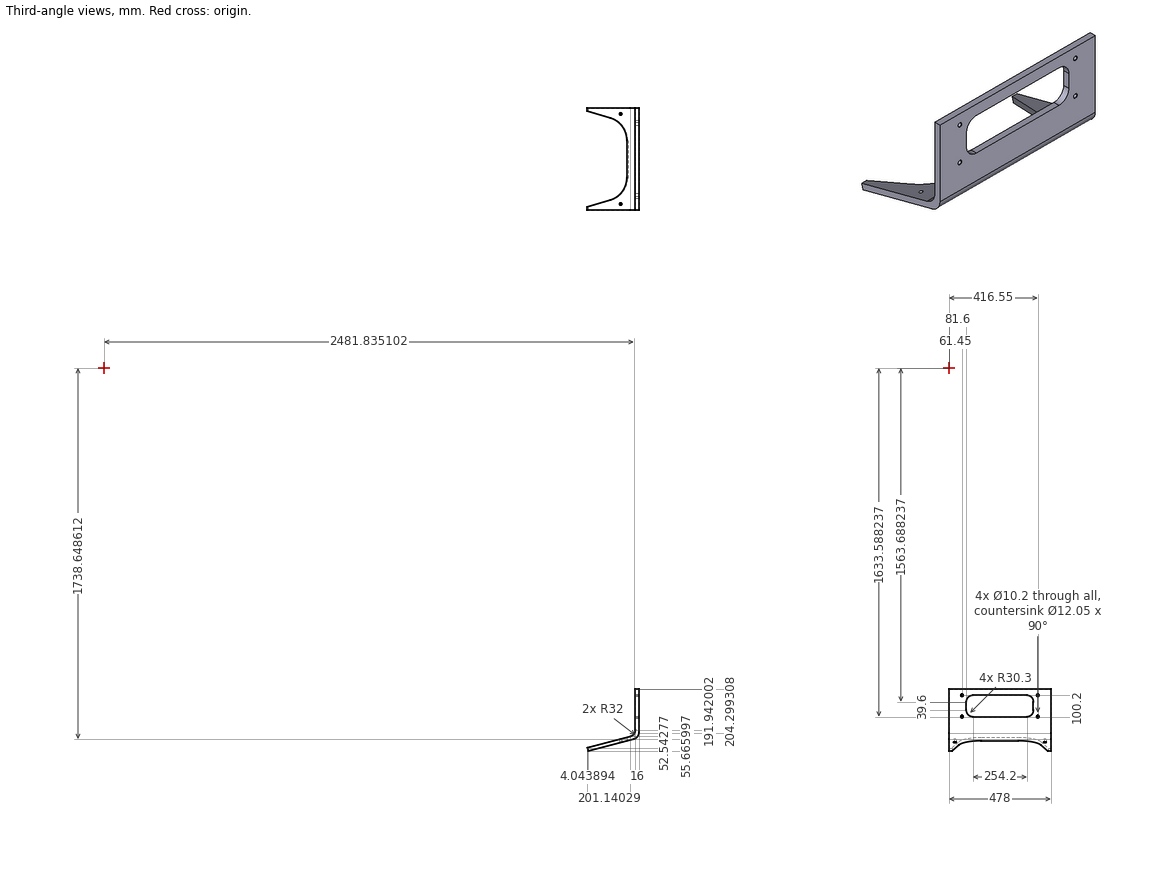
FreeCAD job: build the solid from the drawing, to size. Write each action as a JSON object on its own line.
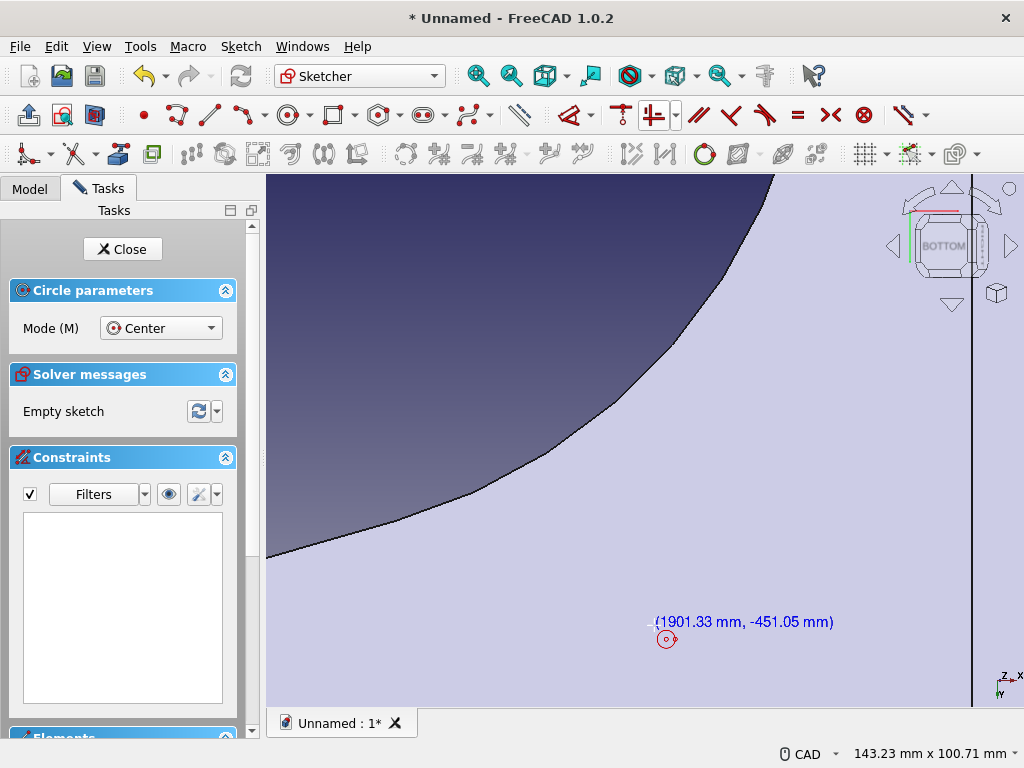
{"action": "scroll", "coordinate": [565, 587], "scroll_direction": "down", "scroll_amount": 10}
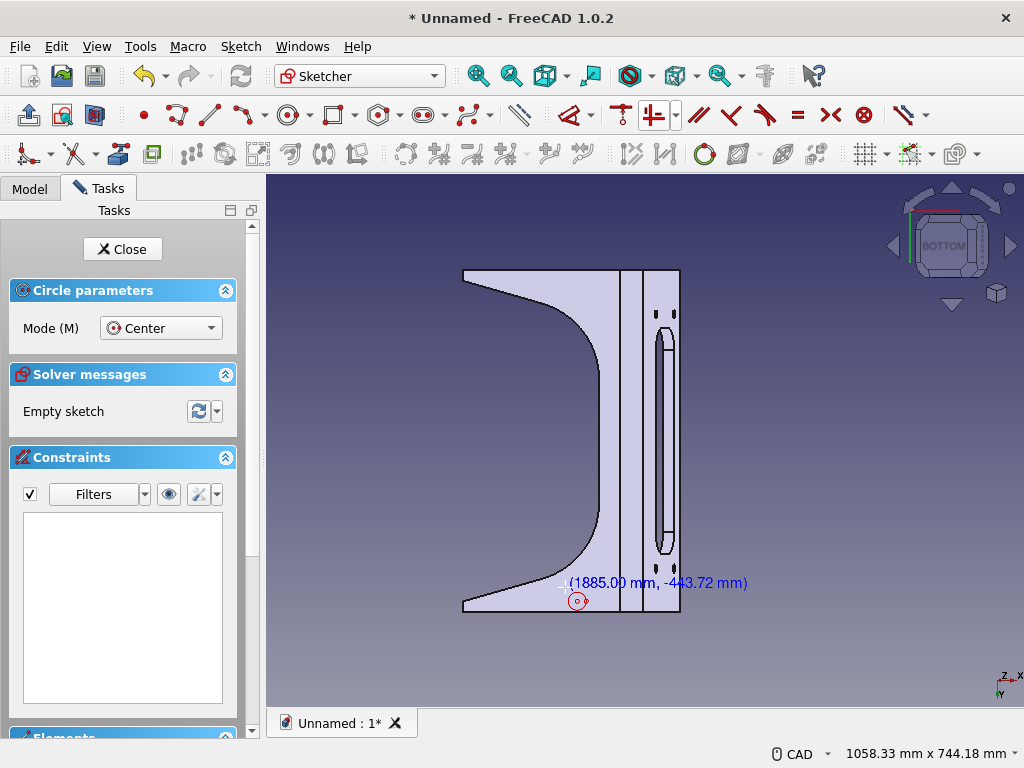
{"action": "left_click", "coordinate": [577, 592]}
{"action": "mouse_move", "coordinate": [580, 590]}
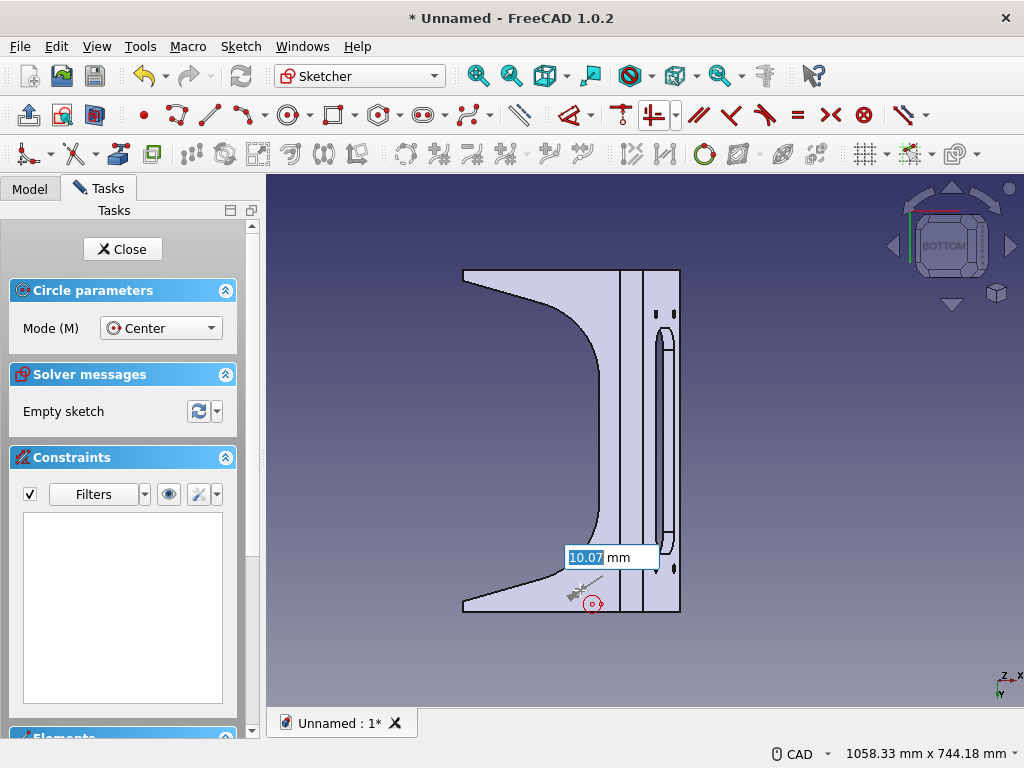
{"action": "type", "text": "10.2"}
{"action": "key", "text": "Return"}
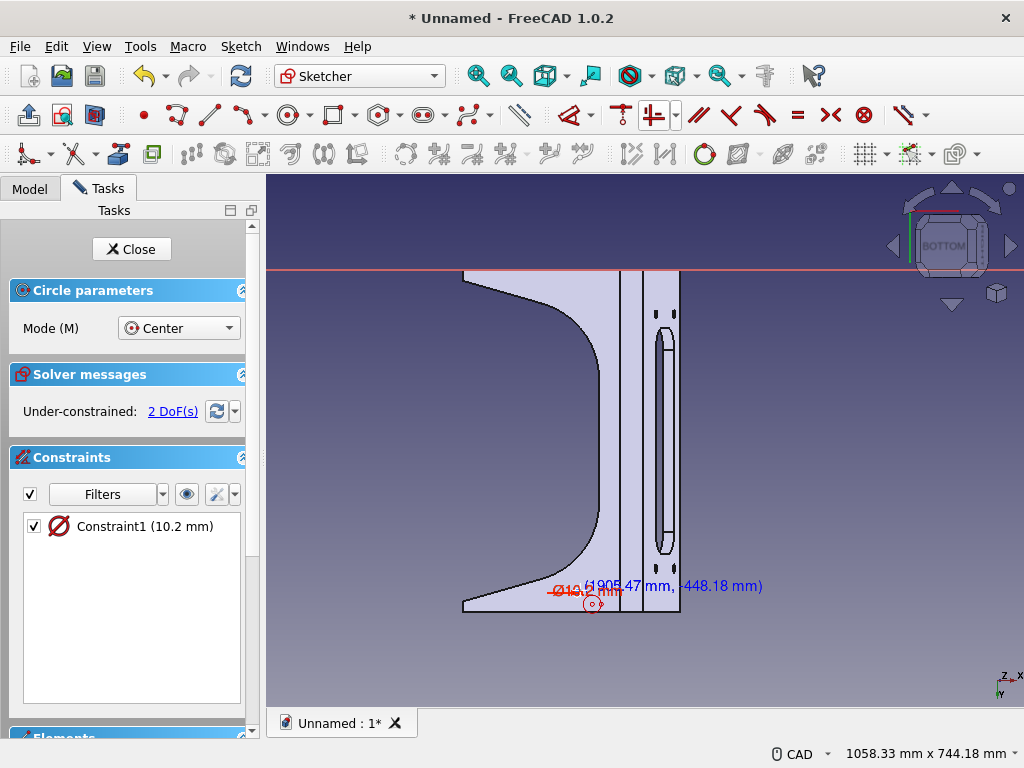
{"action": "scroll", "coordinate": [577, 290], "scroll_direction": "up", "scroll_amount": 10}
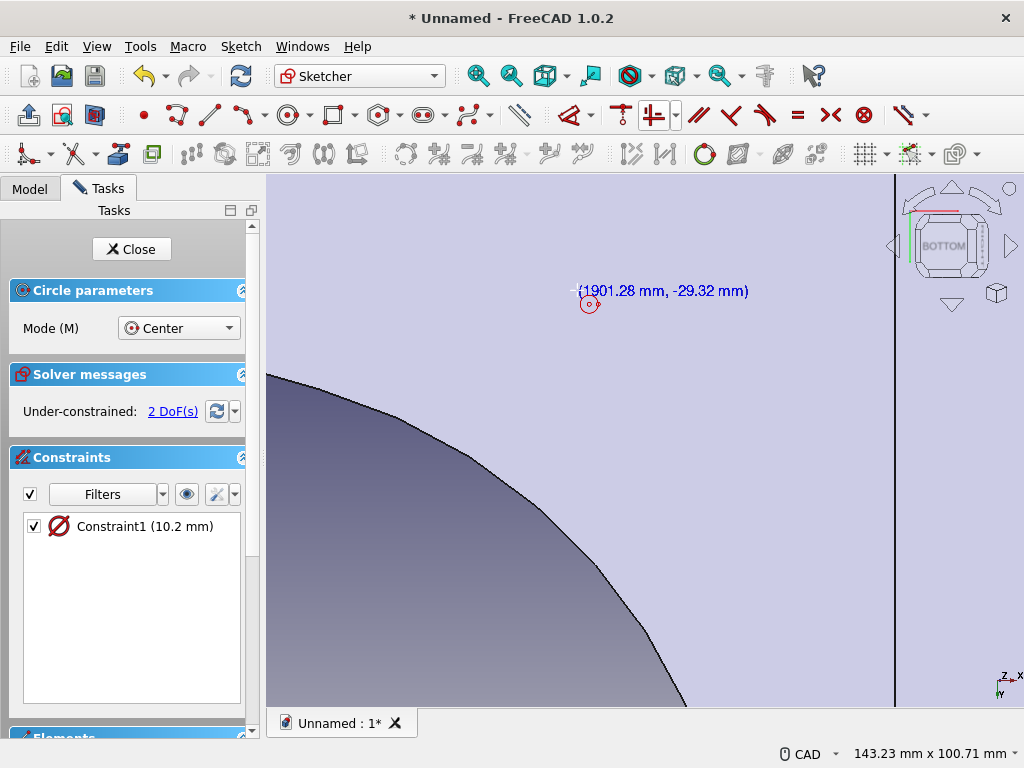
{"action": "scroll", "coordinate": [577, 289], "scroll_direction": "down", "scroll_amount": 10}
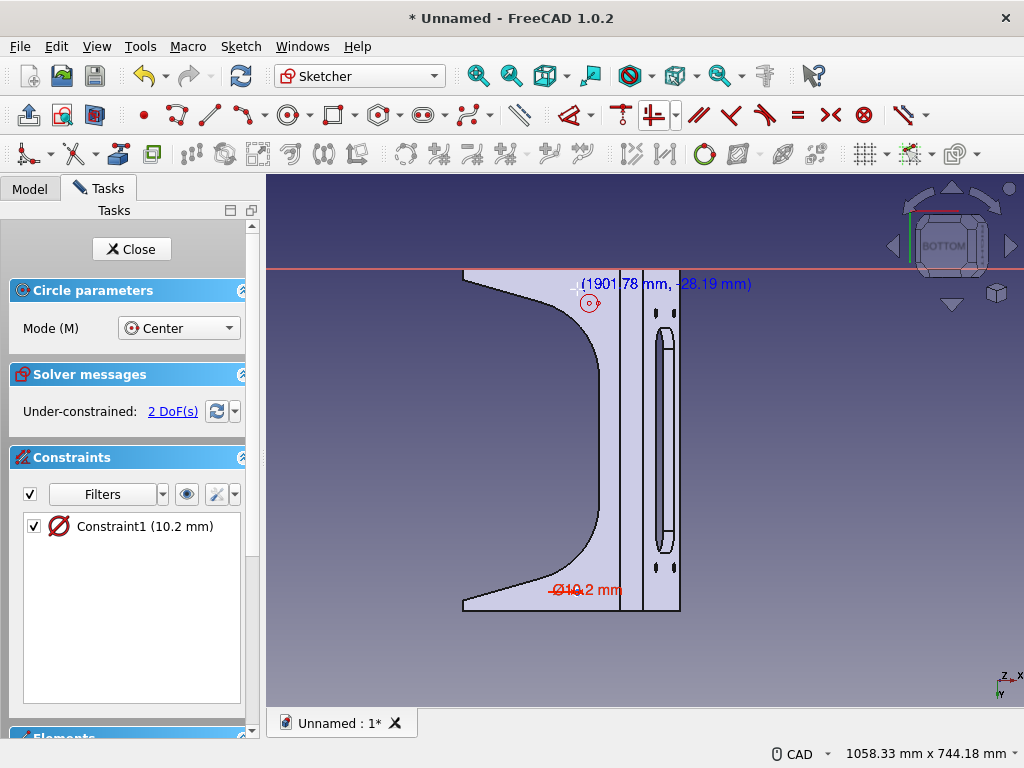
{"action": "left_click", "coordinate": [577, 289]}
{"action": "mouse_move", "coordinate": [580, 287]}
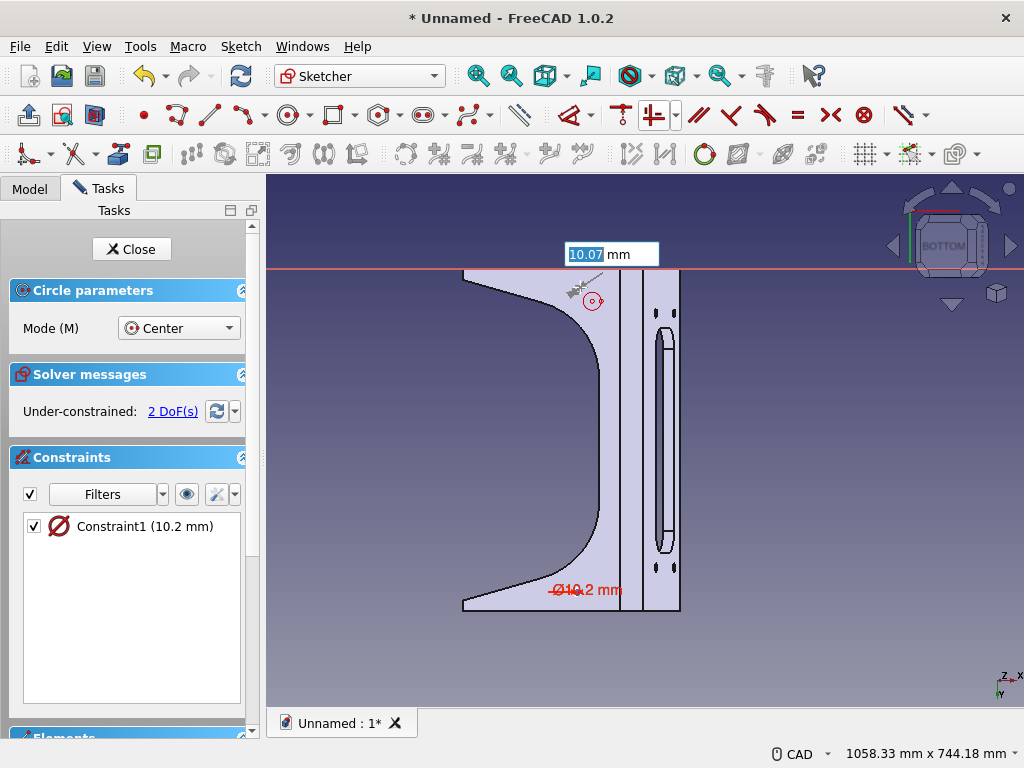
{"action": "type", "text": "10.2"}
{"action": "key", "text": "Return"}
{"action": "key", "text": "Escape"}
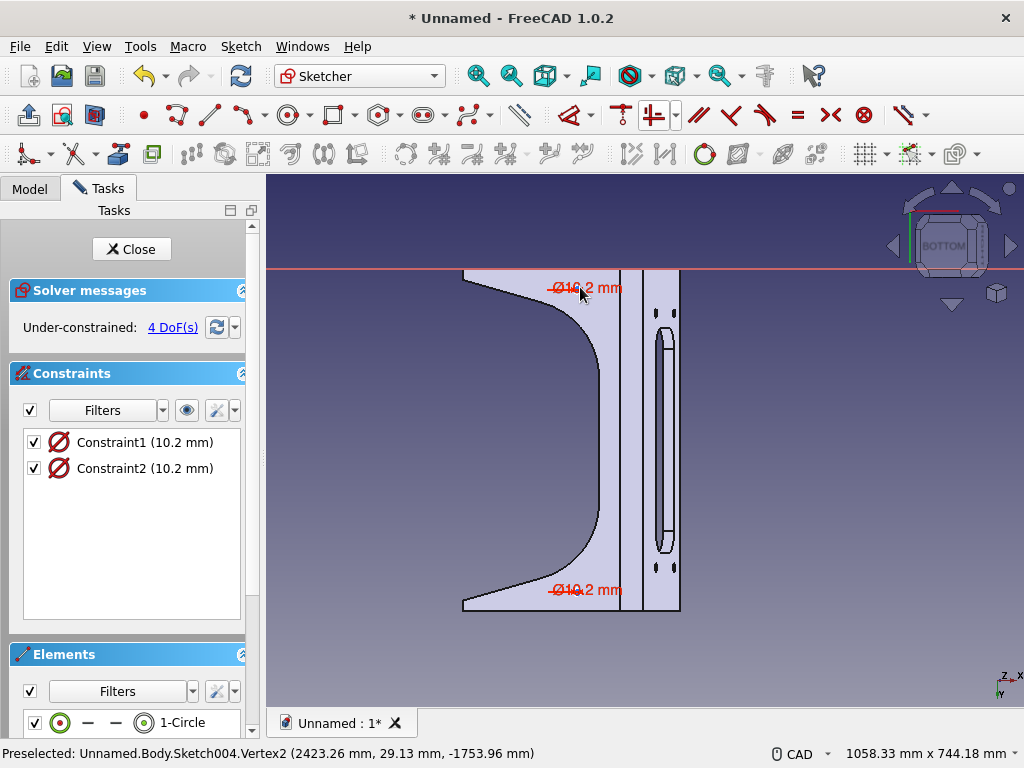
{"action": "left_click", "coordinate": [568, 116]}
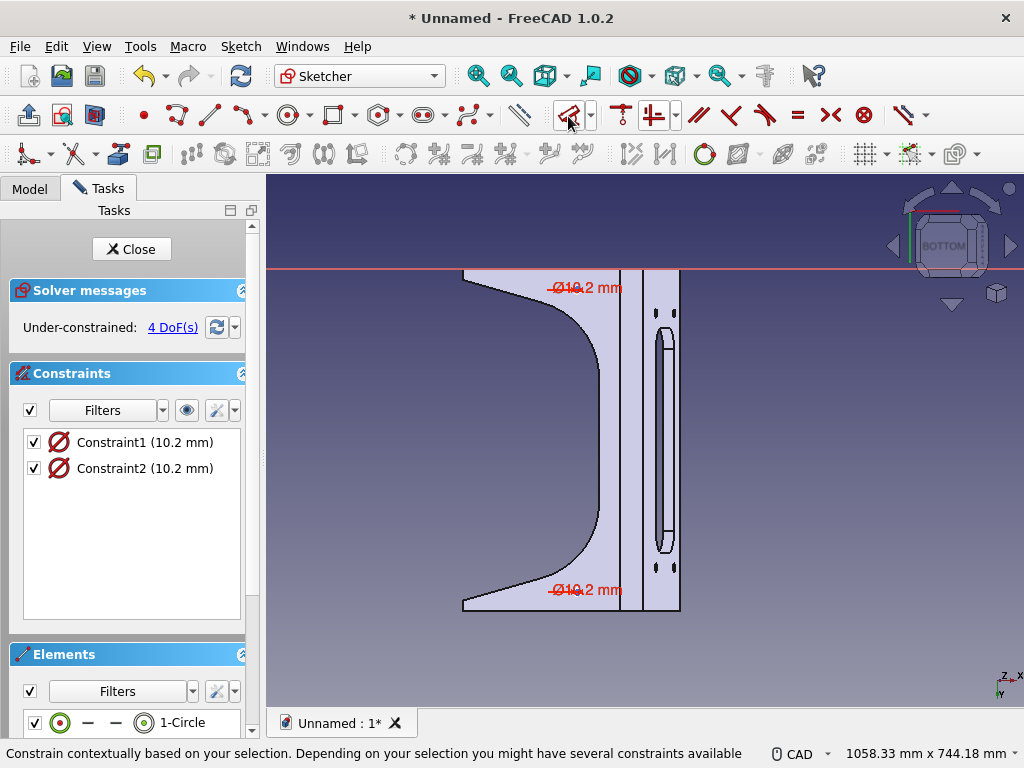
{"action": "scroll", "coordinate": [577, 290], "scroll_direction": "up", "scroll_amount": 4}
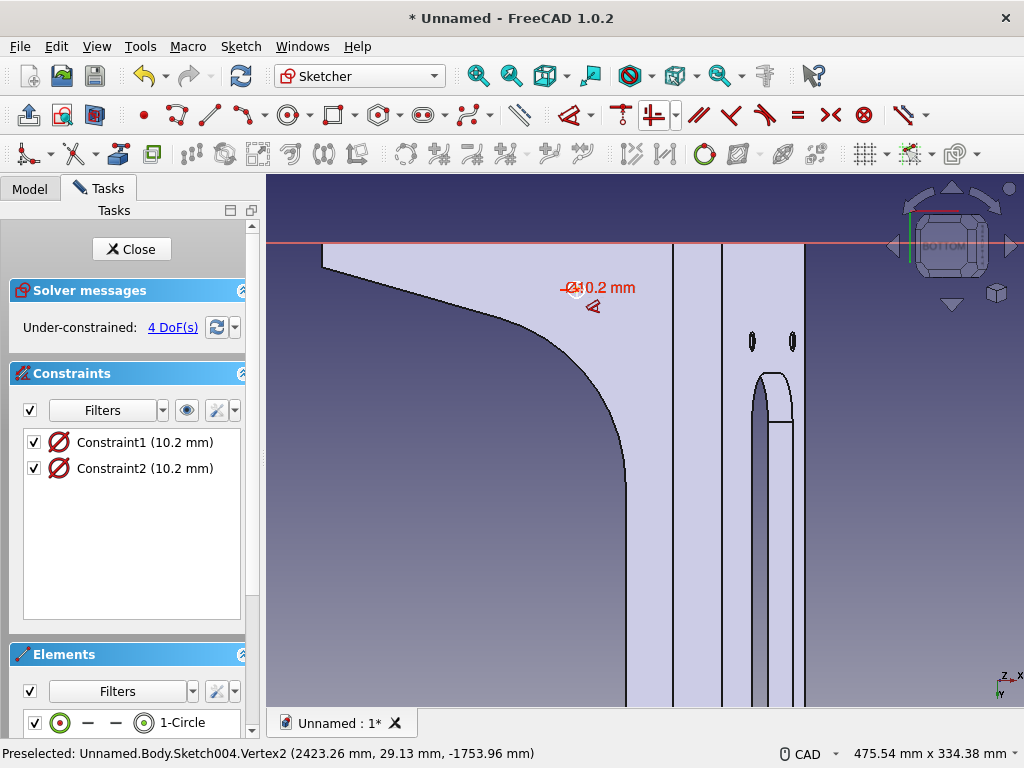
{"action": "left_click", "coordinate": [576, 290]}
{"action": "left_click", "coordinate": [610, 267]}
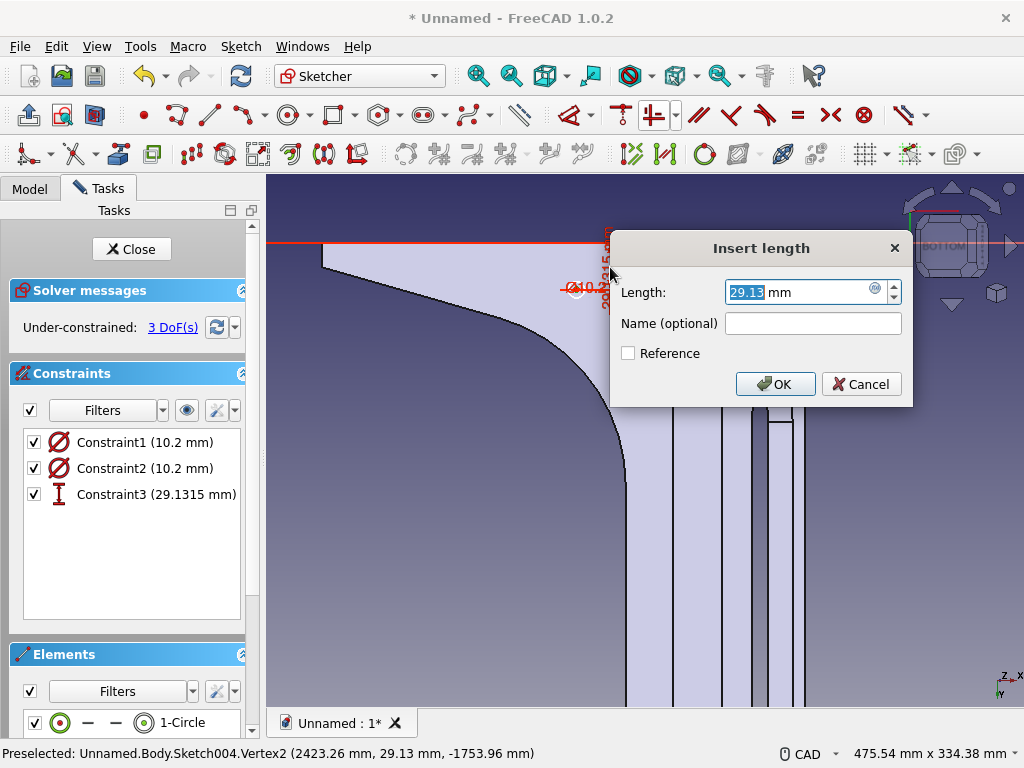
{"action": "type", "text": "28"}
{"action": "key", "text": "Return"}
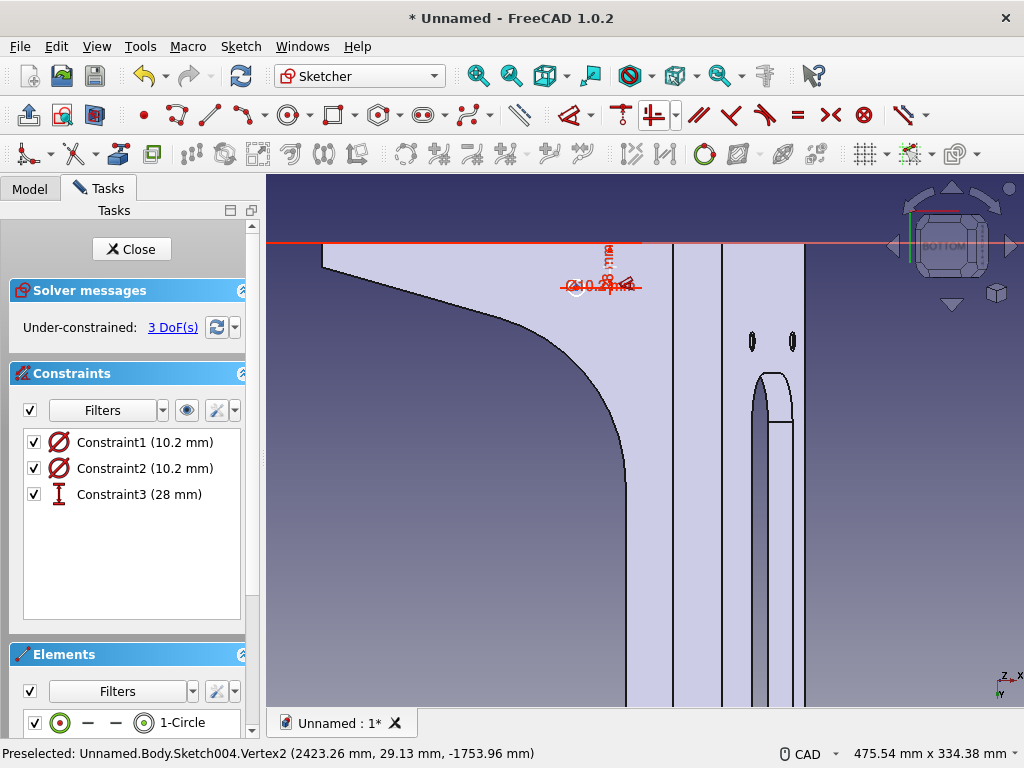
{"action": "scroll", "coordinate": [576, 291], "scroll_direction": "down", "scroll_amount": 4}